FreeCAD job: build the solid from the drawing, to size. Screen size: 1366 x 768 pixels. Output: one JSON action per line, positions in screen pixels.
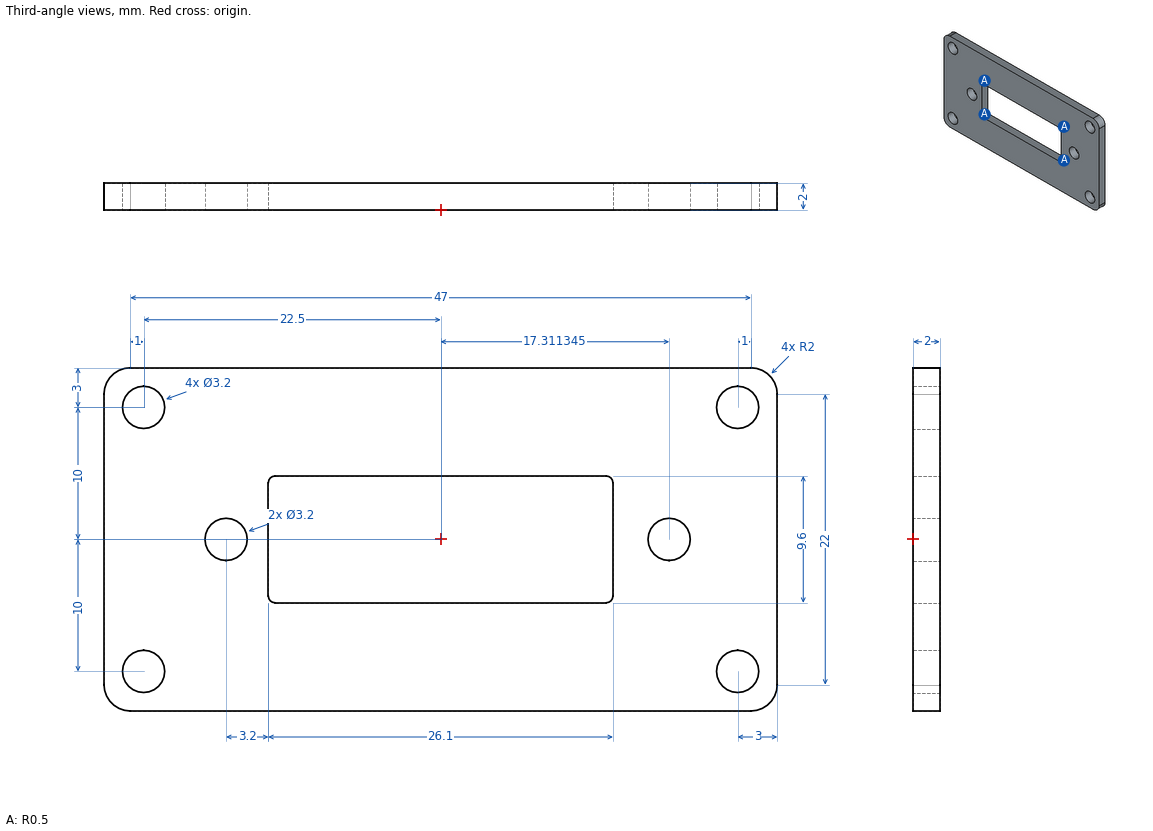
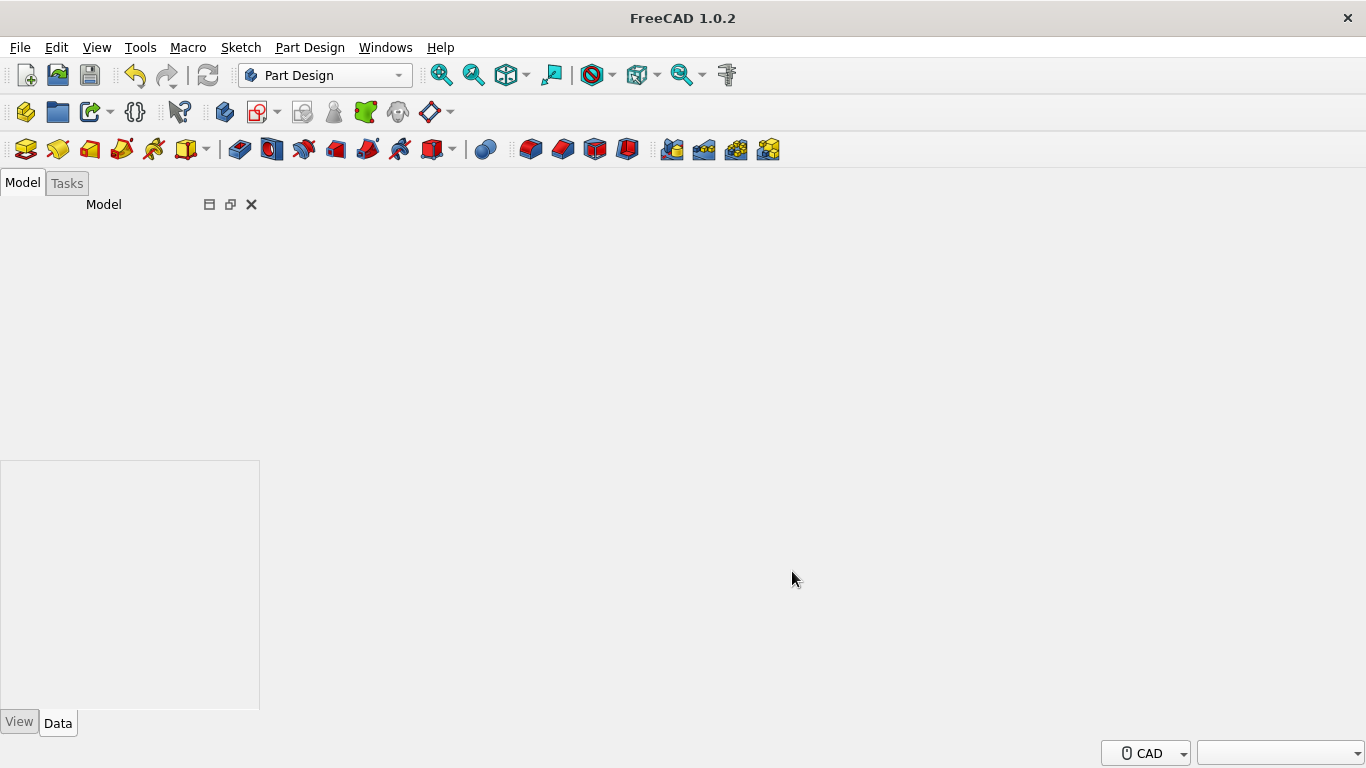
{"action": "left_click", "coordinate": [26, 76]}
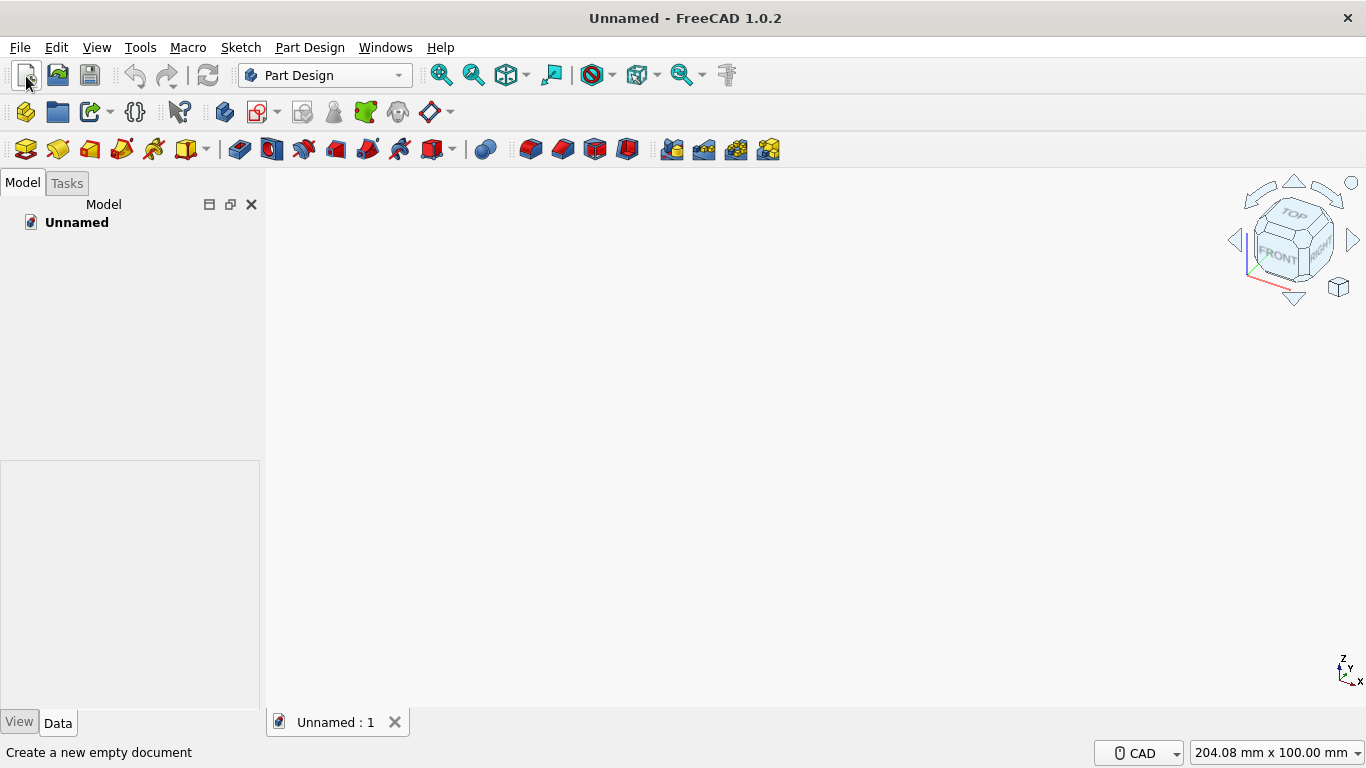
{"action": "left_click", "coordinate": [258, 112]}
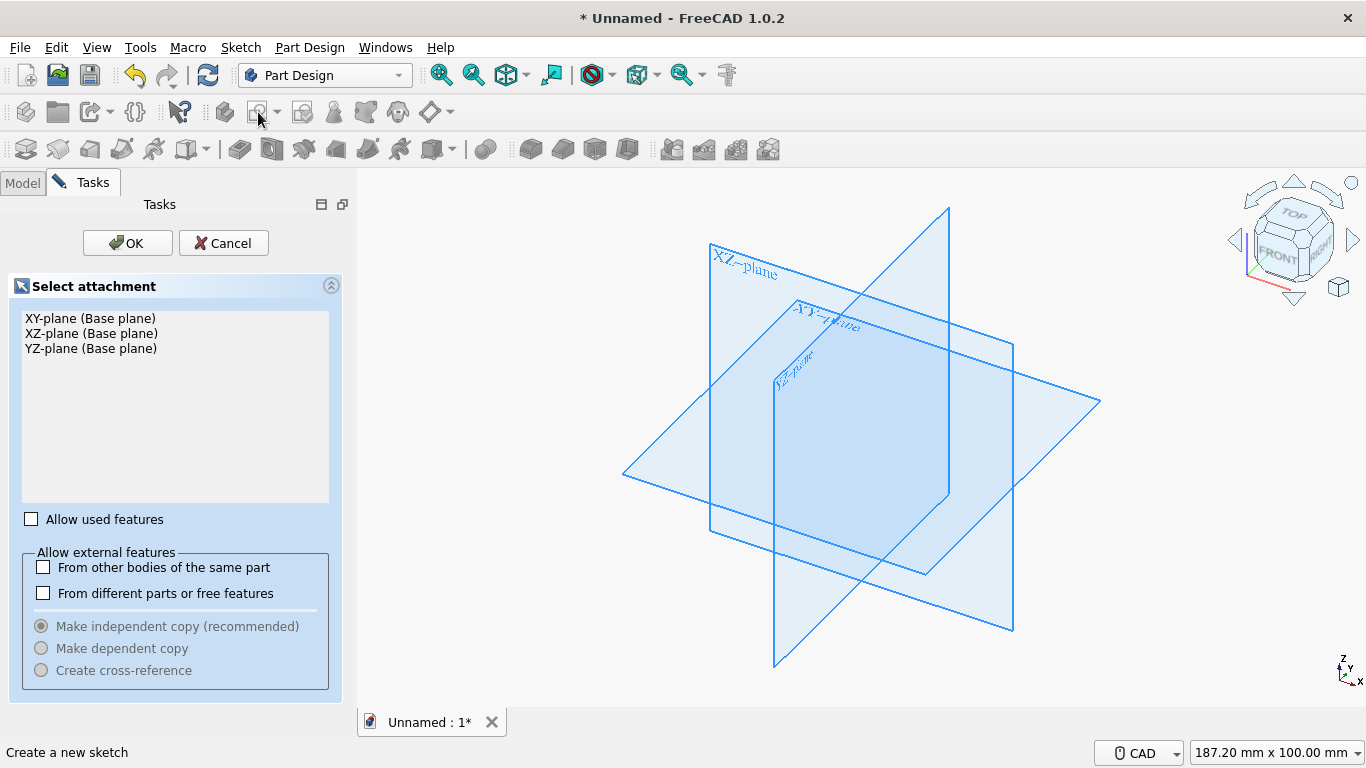
{"action": "left_click", "coordinate": [82, 334]}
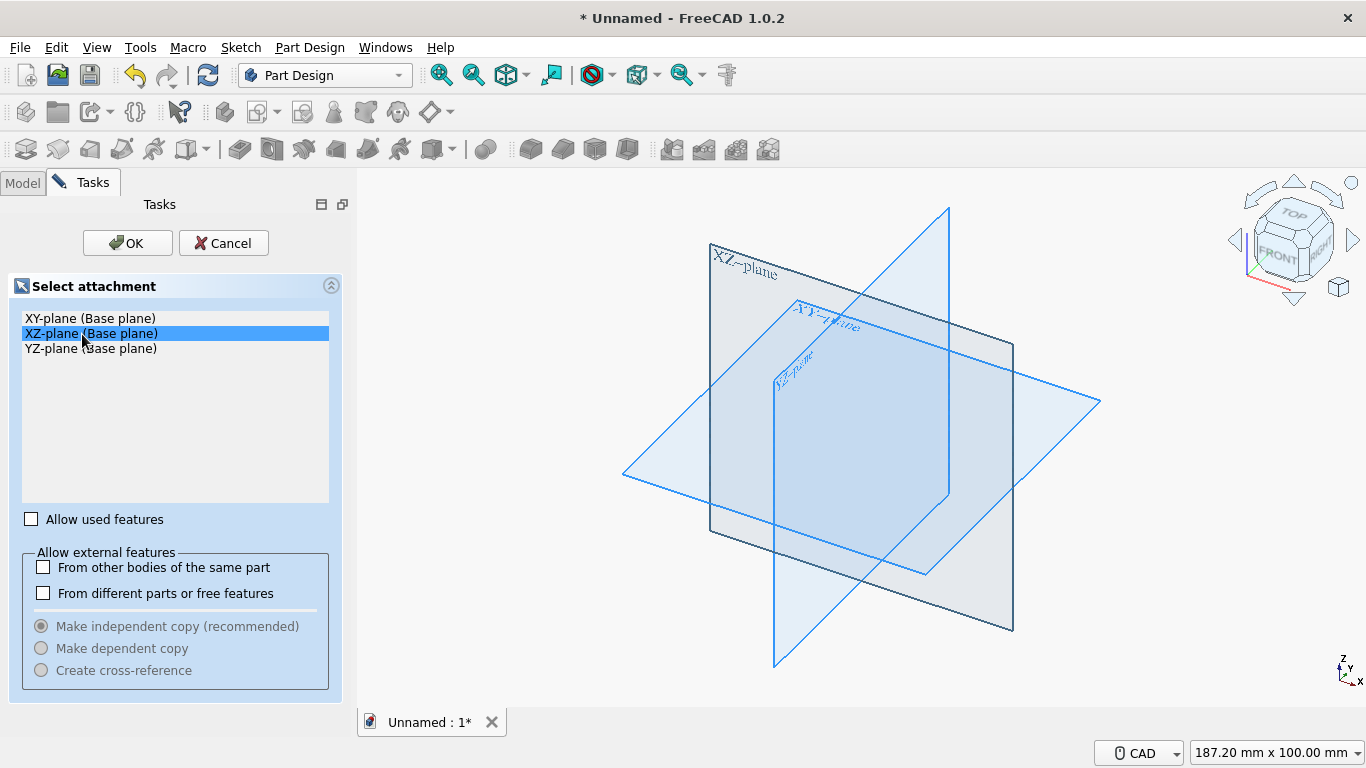
{"action": "left_click", "coordinate": [128, 243]}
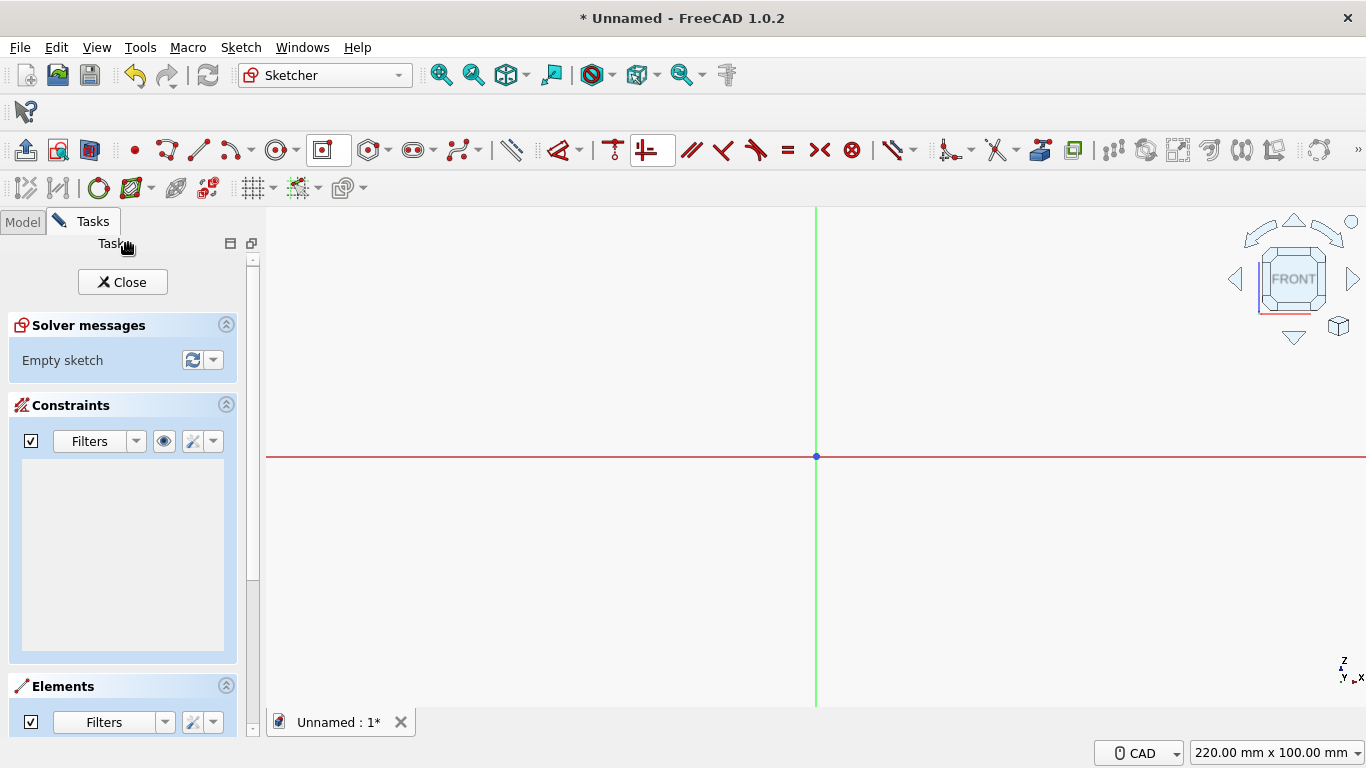
{"action": "scroll", "coordinate": [872, 457], "scroll_direction": "up", "scroll_amount": 4}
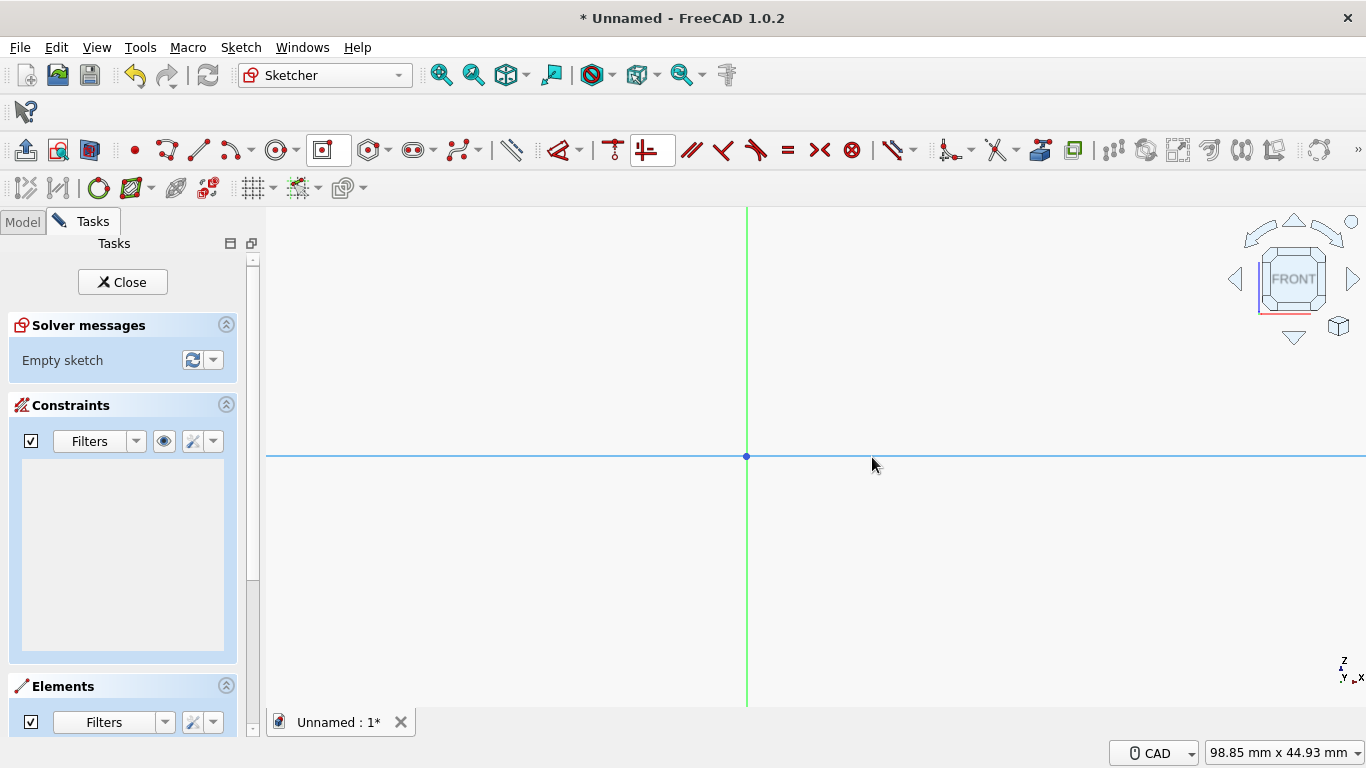
{"action": "left_click", "coordinate": [200, 150]}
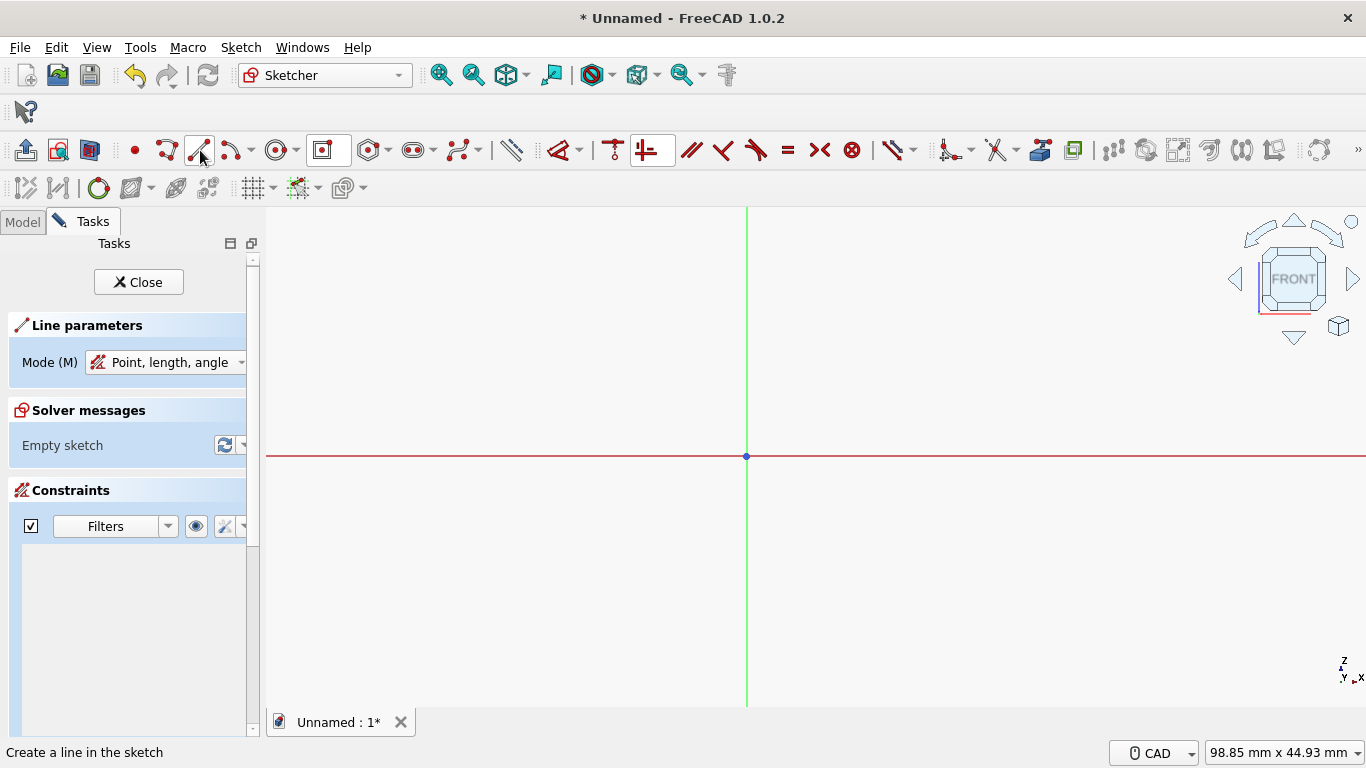
{"action": "left_click", "coordinate": [485, 312]}
{"action": "left_click", "coordinate": [1008, 312]}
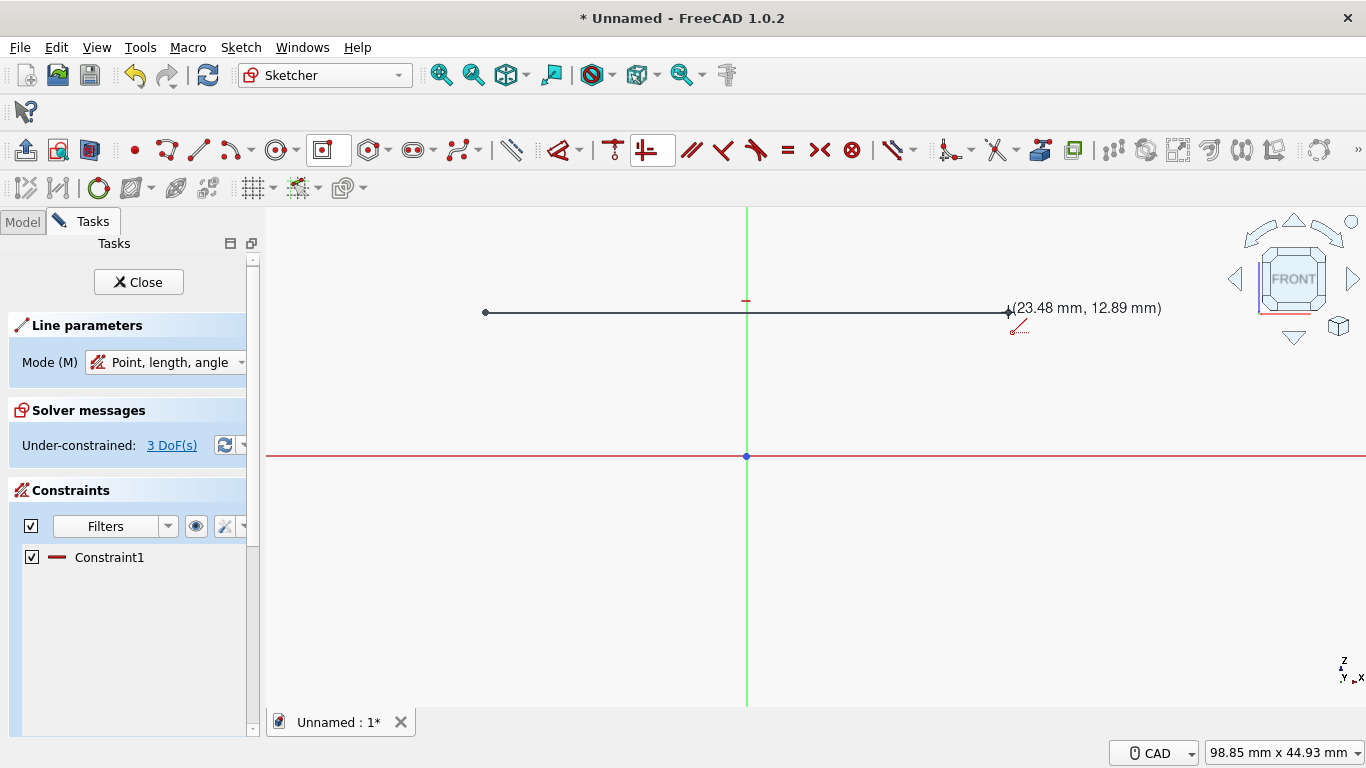
{"action": "left_click", "coordinate": [1030, 334]}
{"action": "left_click", "coordinate": [1030, 579]}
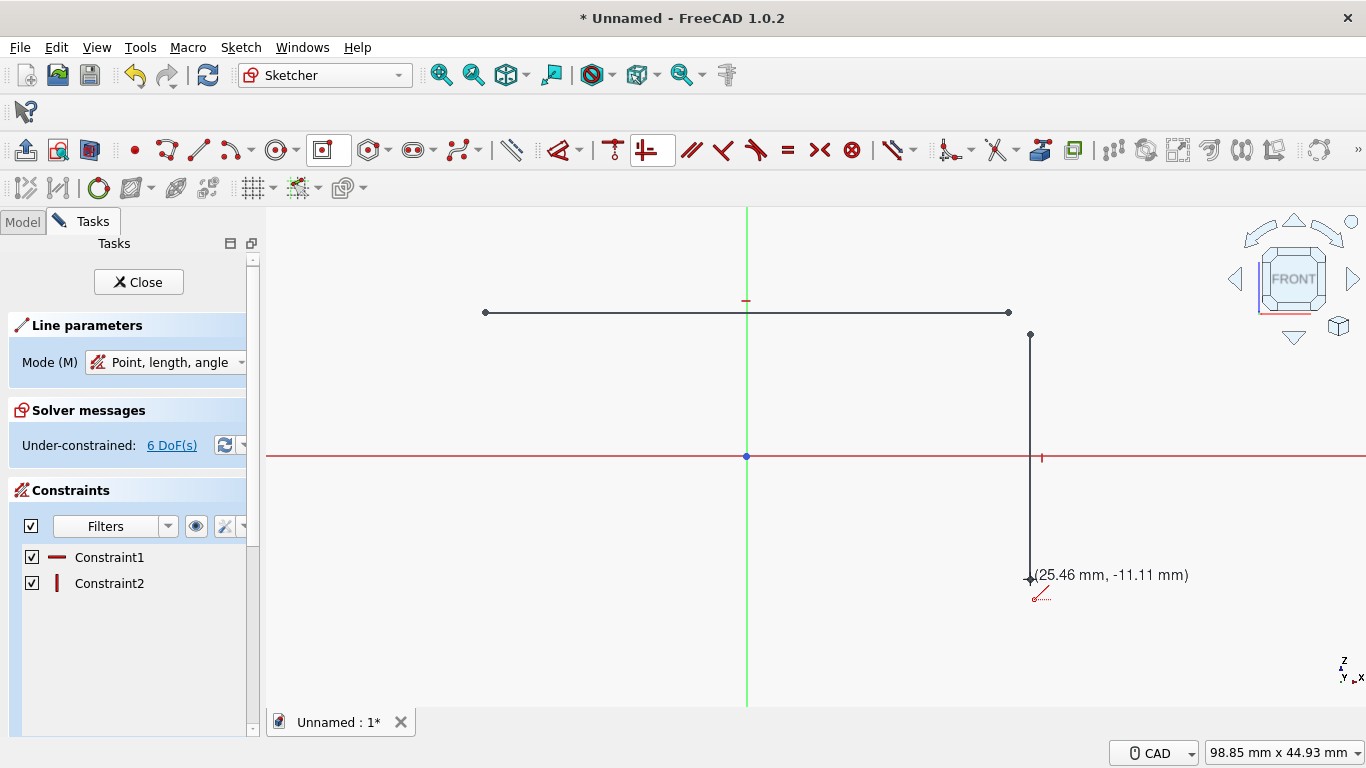
{"action": "left_click", "coordinate": [1008, 601]}
{"action": "left_click", "coordinate": [485, 601]}